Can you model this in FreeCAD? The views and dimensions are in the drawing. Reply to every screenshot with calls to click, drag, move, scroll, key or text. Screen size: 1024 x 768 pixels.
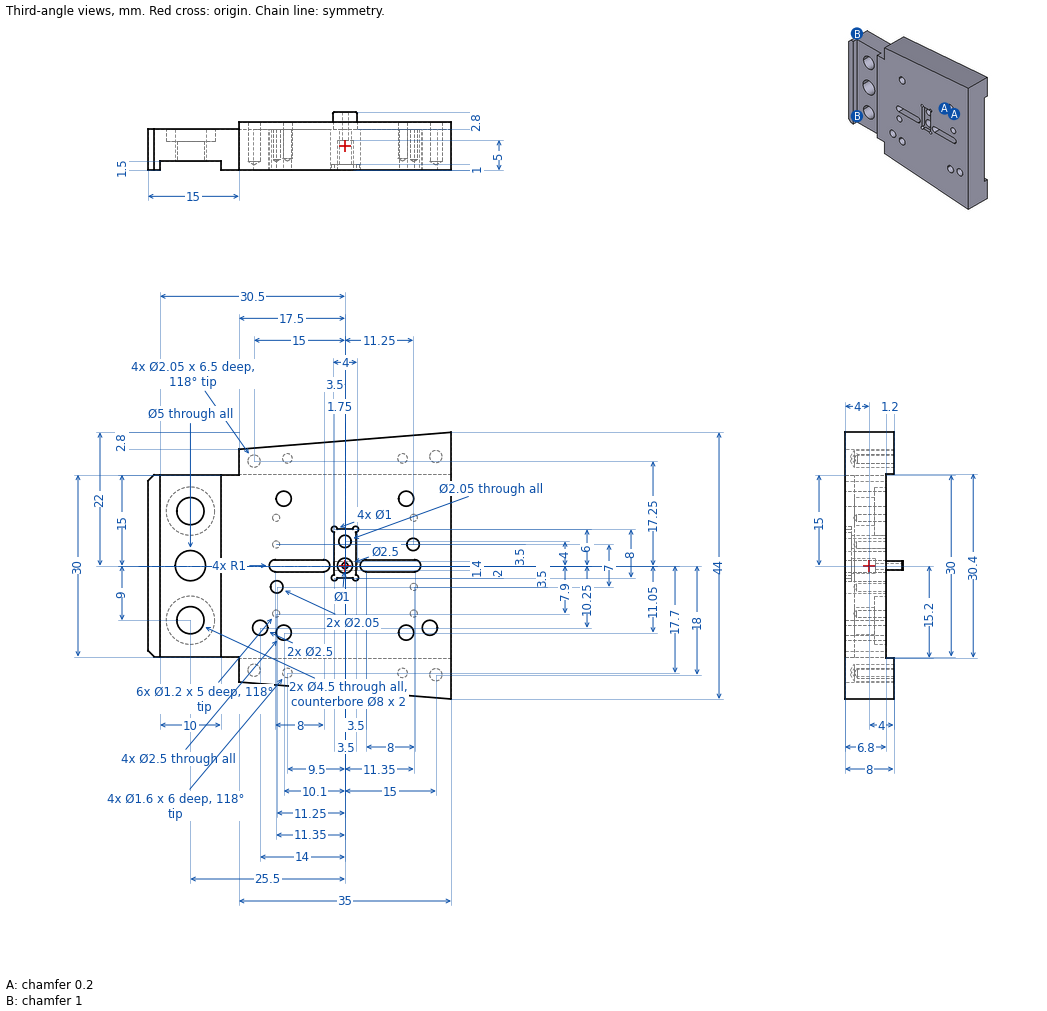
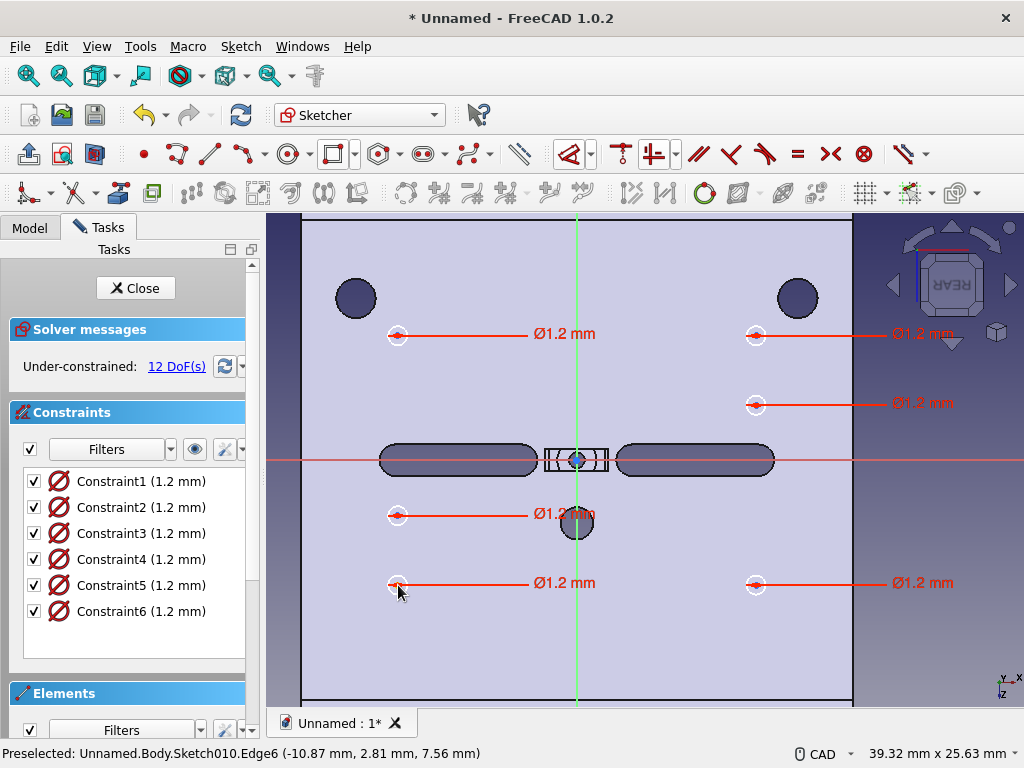
click(398, 336)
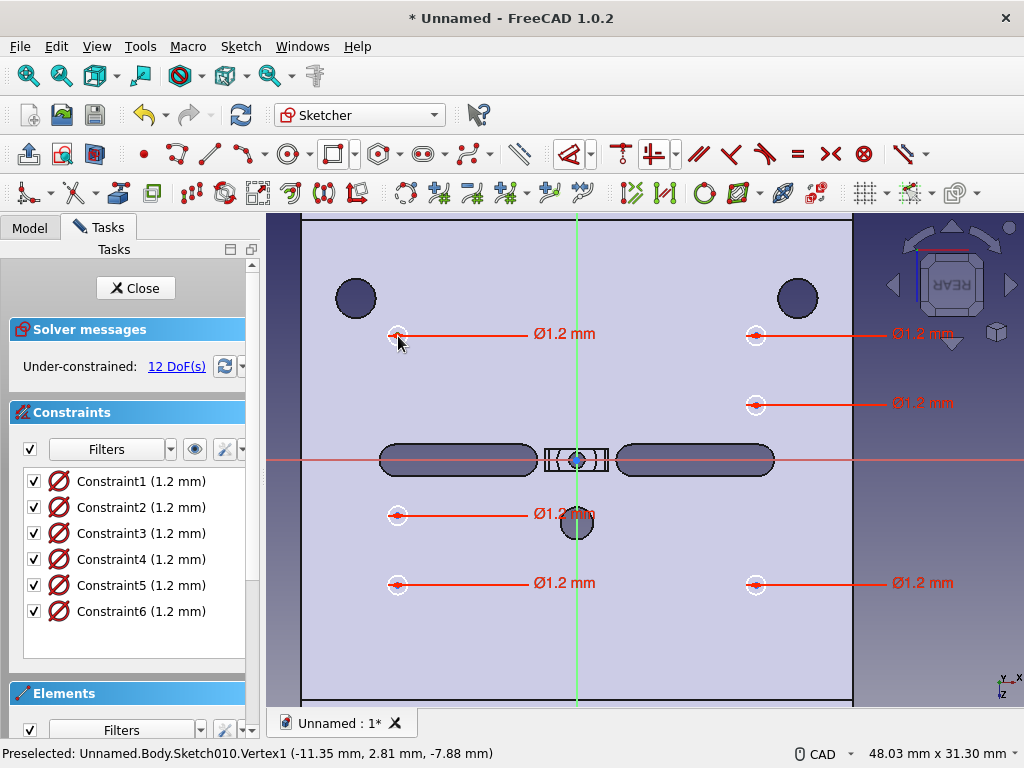
click(756, 336)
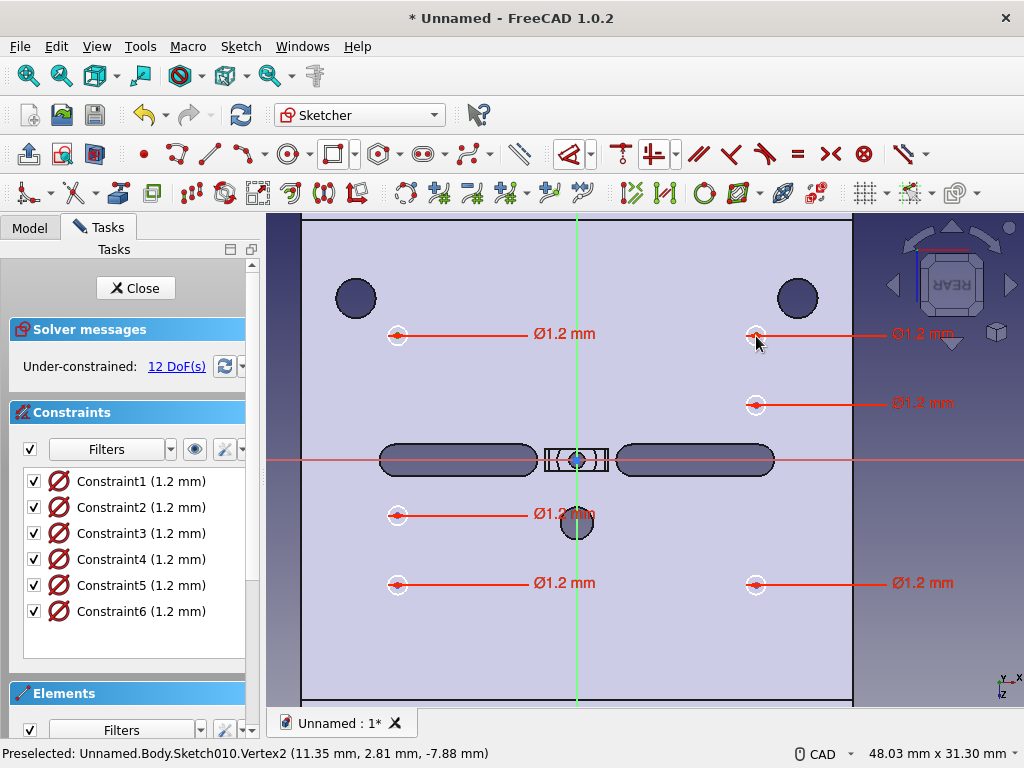
click(577, 648)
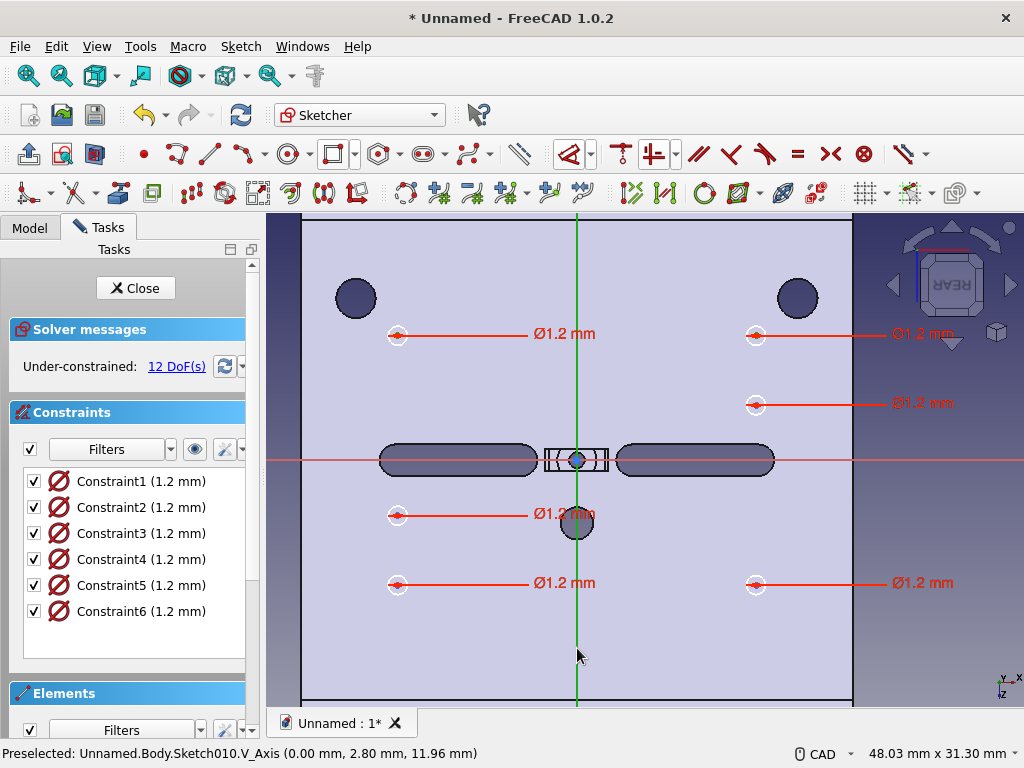
click(831, 154)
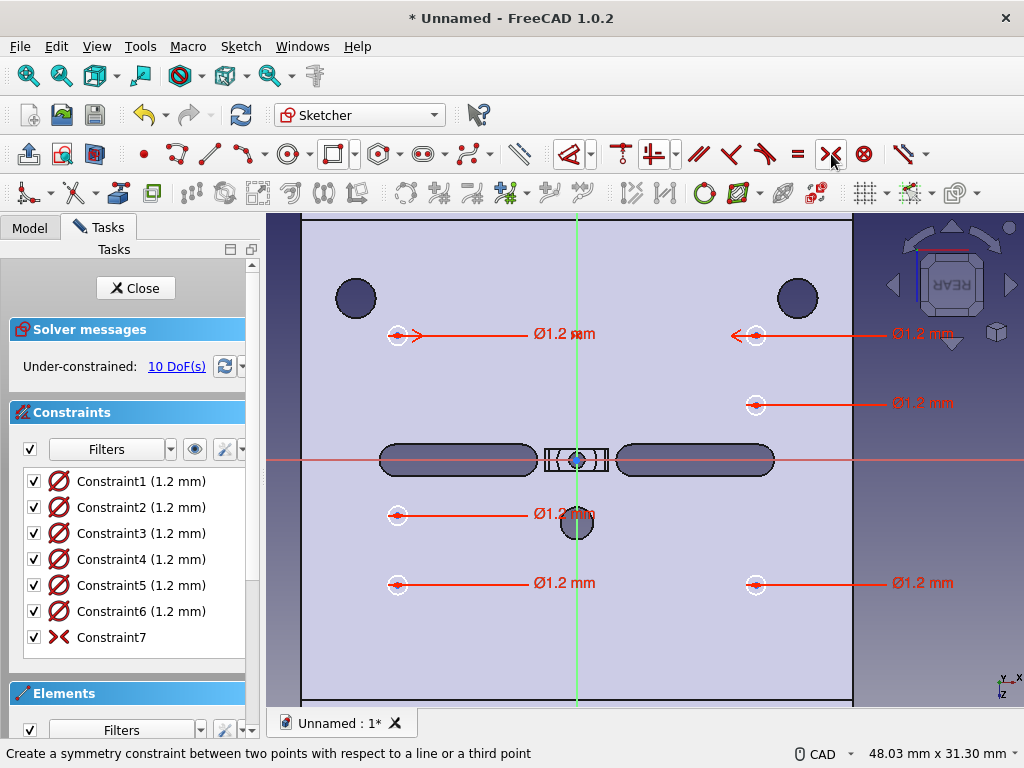
click(756, 336)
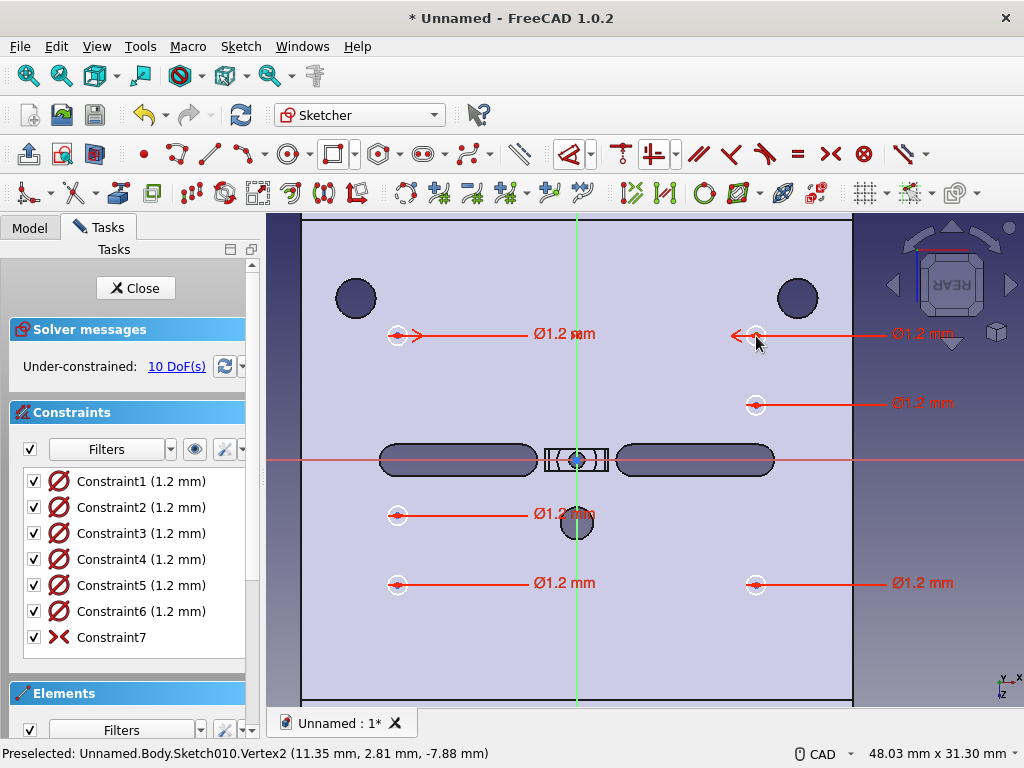
click(756, 585)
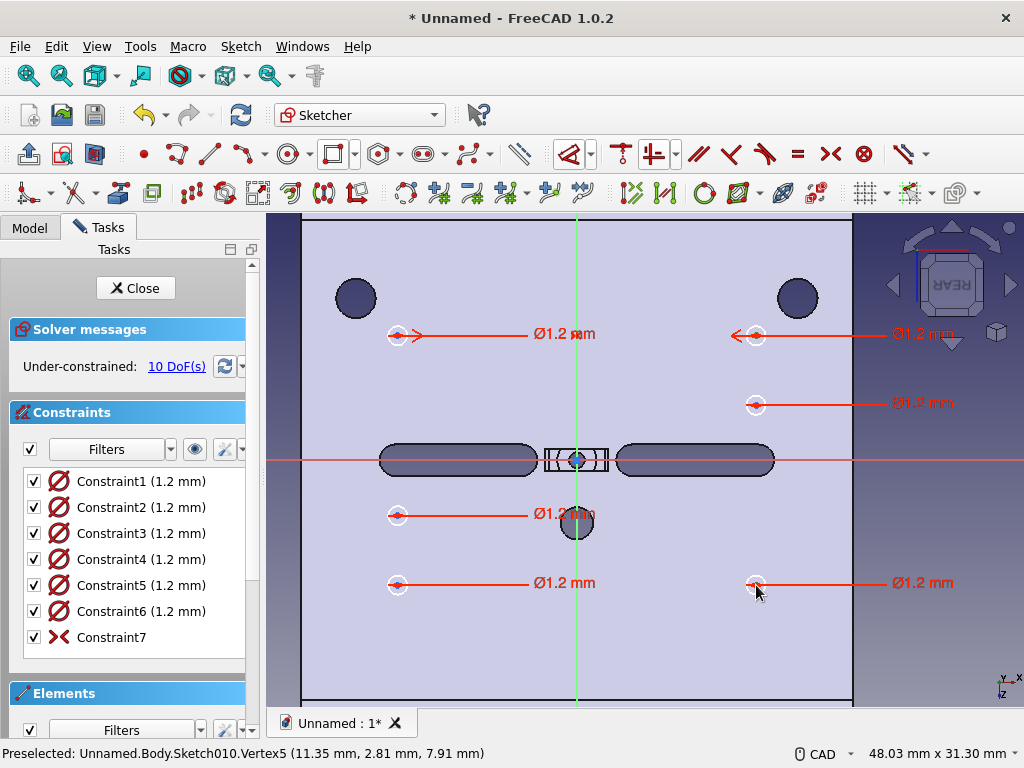
click(334, 460)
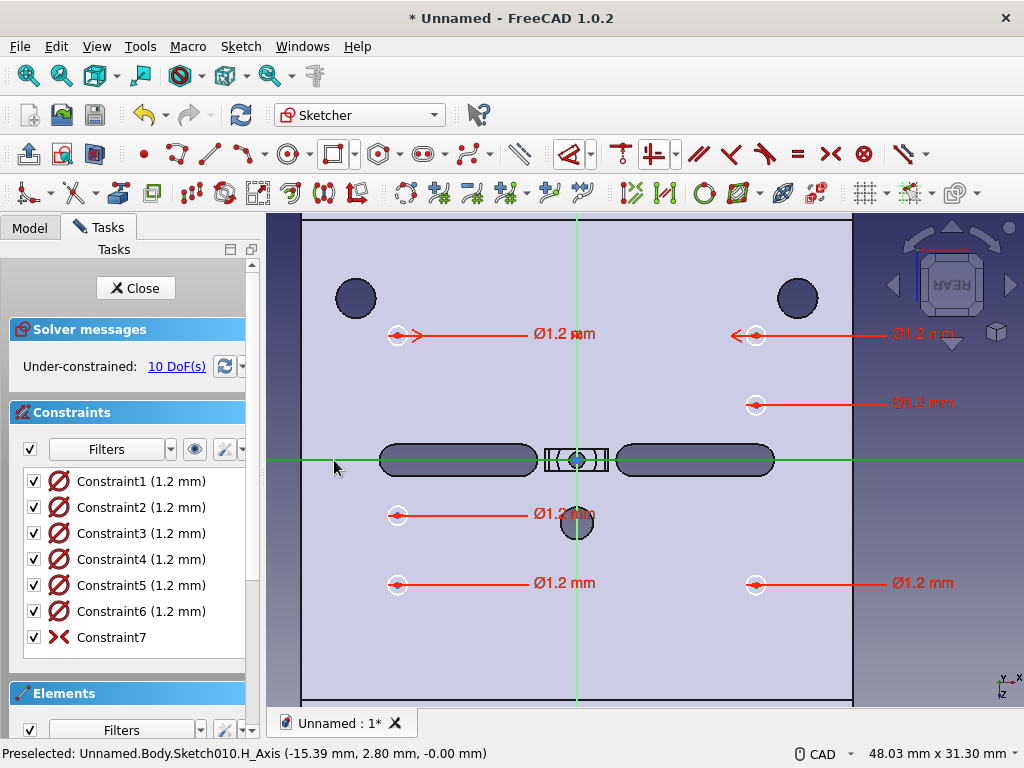
click(831, 154)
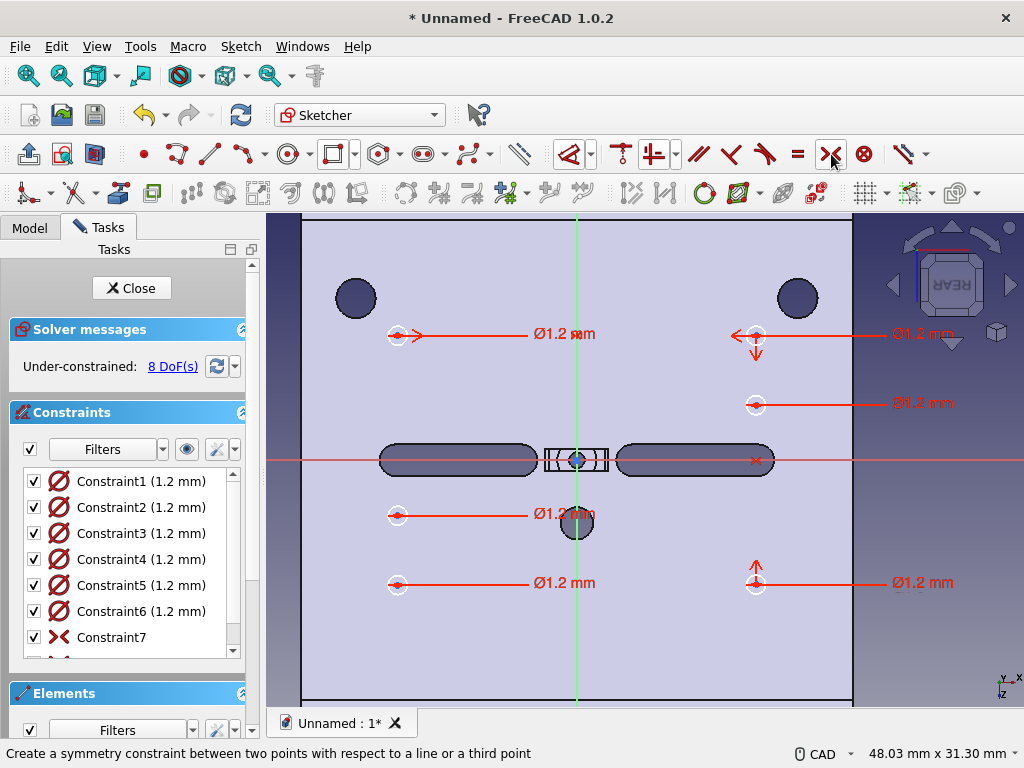
click(398, 336)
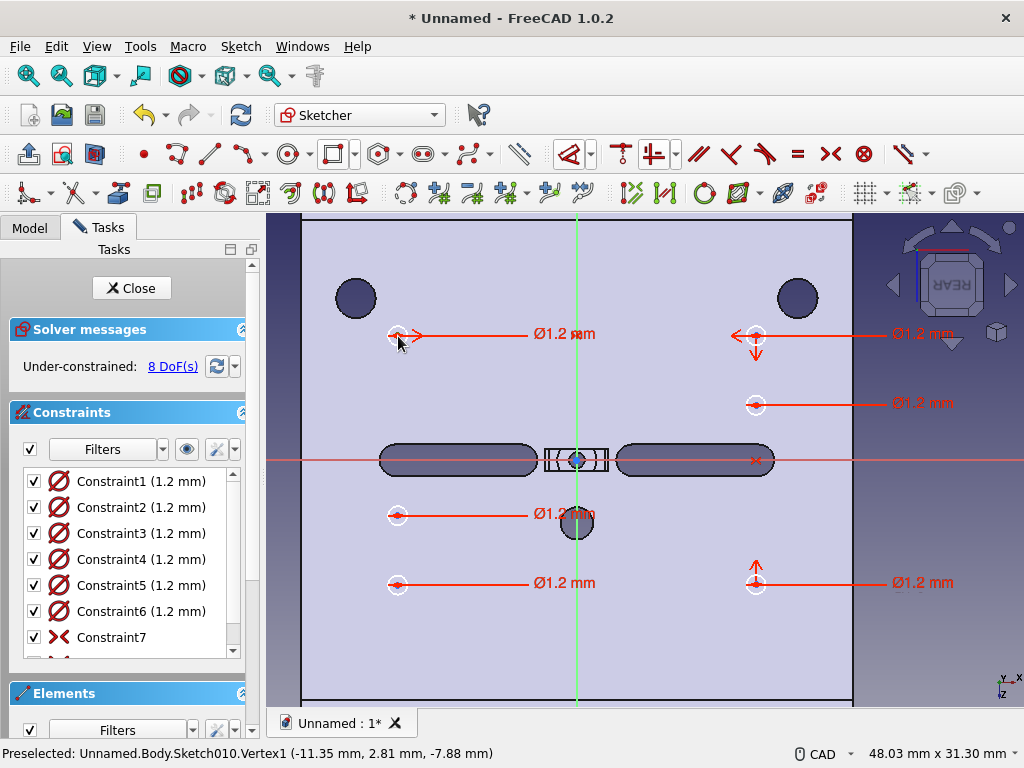
click(398, 585)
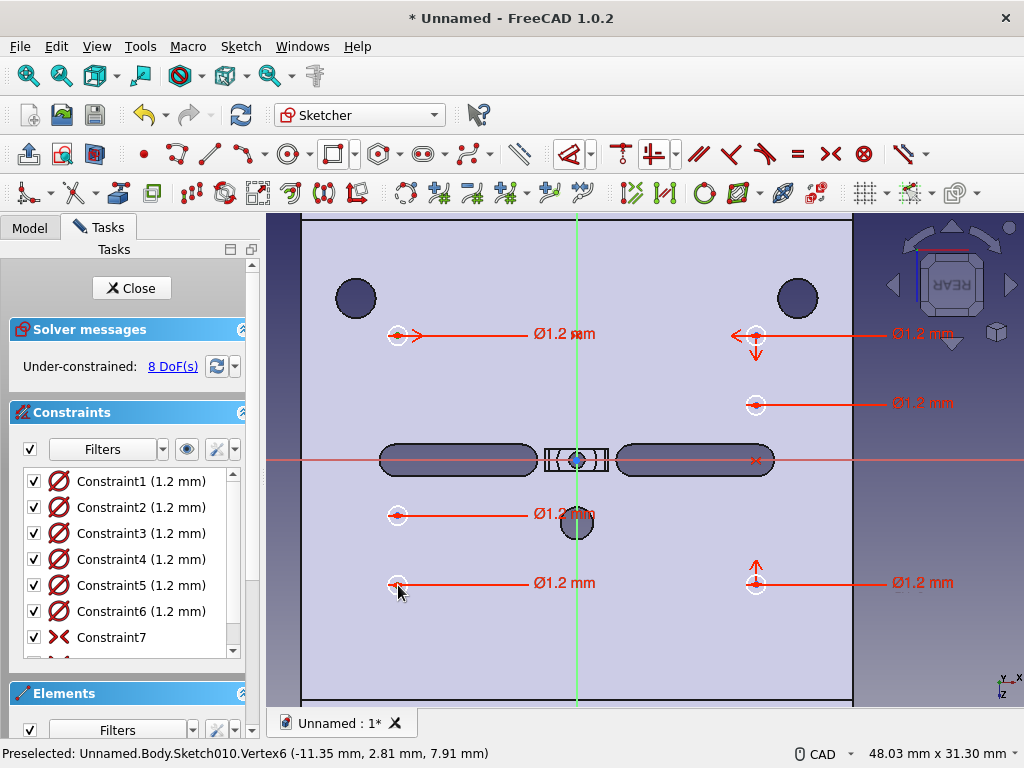
click(334, 460)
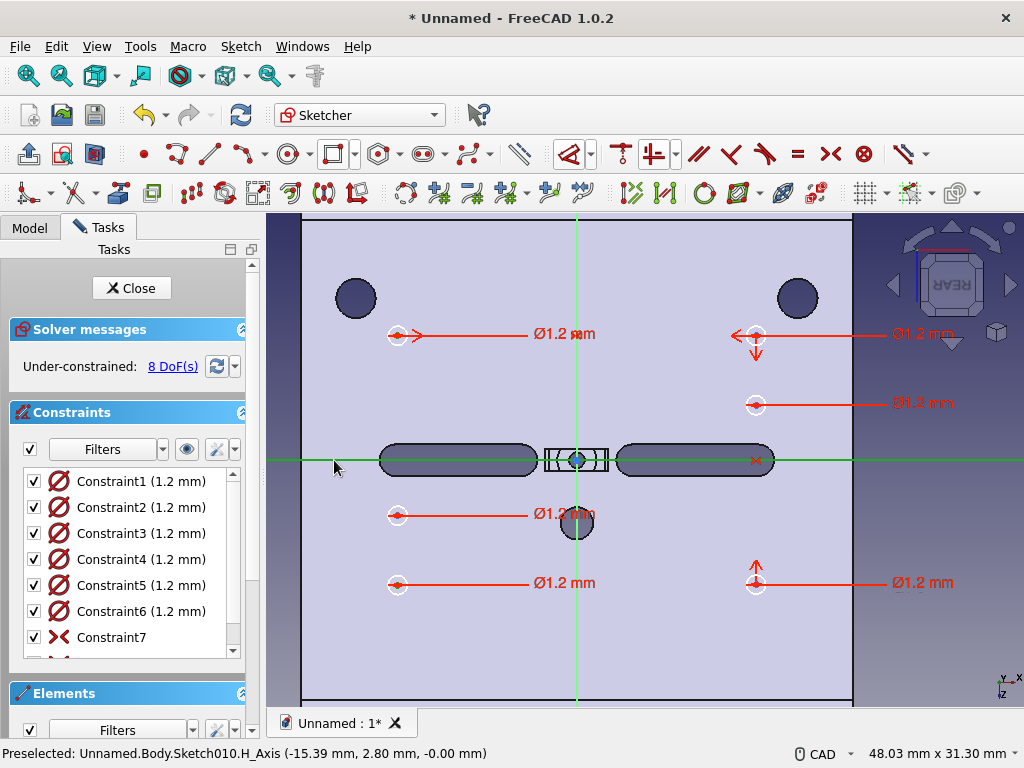
click(831, 154)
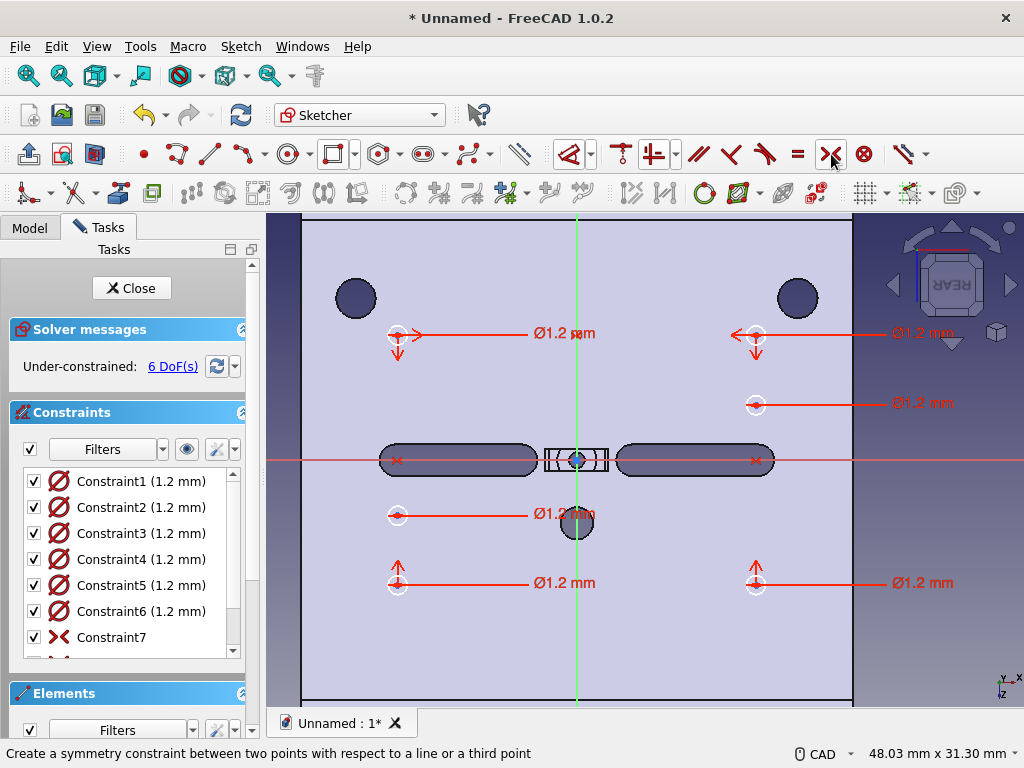
click(398, 516)